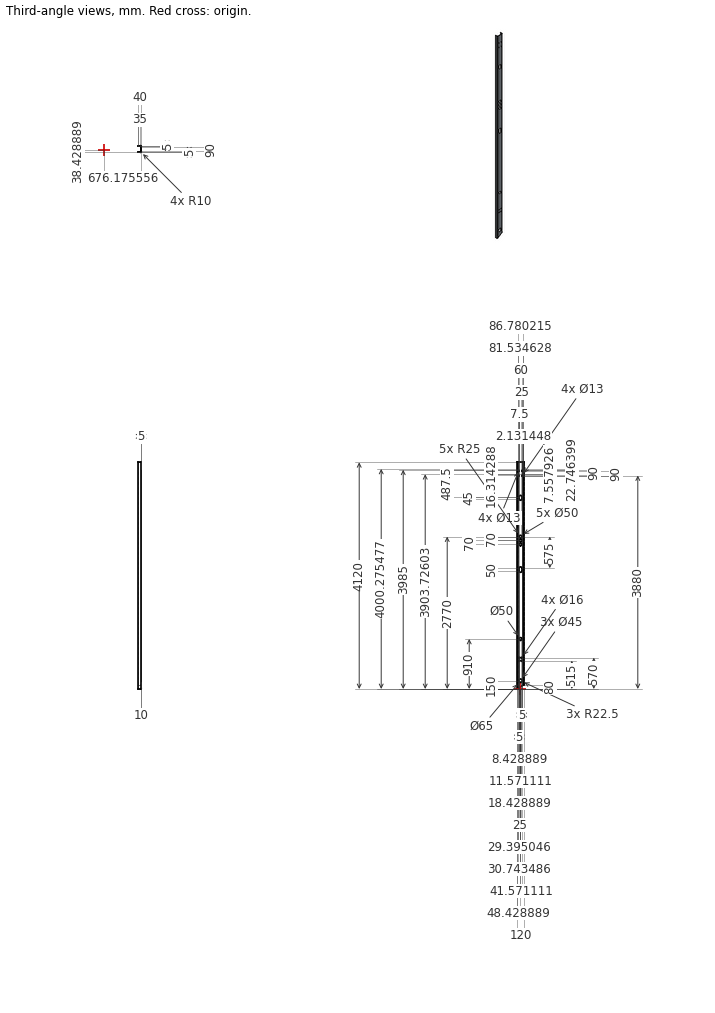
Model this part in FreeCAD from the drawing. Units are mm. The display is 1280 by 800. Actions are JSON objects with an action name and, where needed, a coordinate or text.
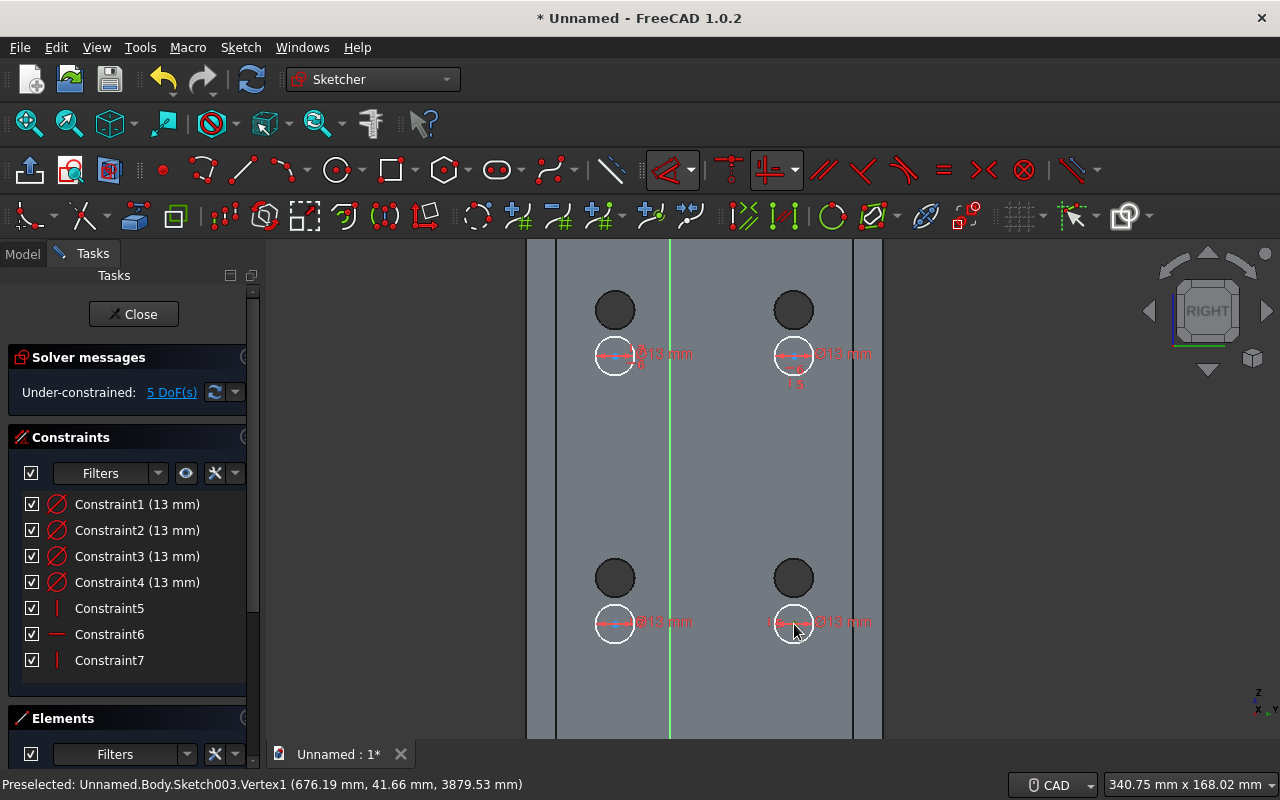
{"action": "left_click", "coordinate": [615, 624]}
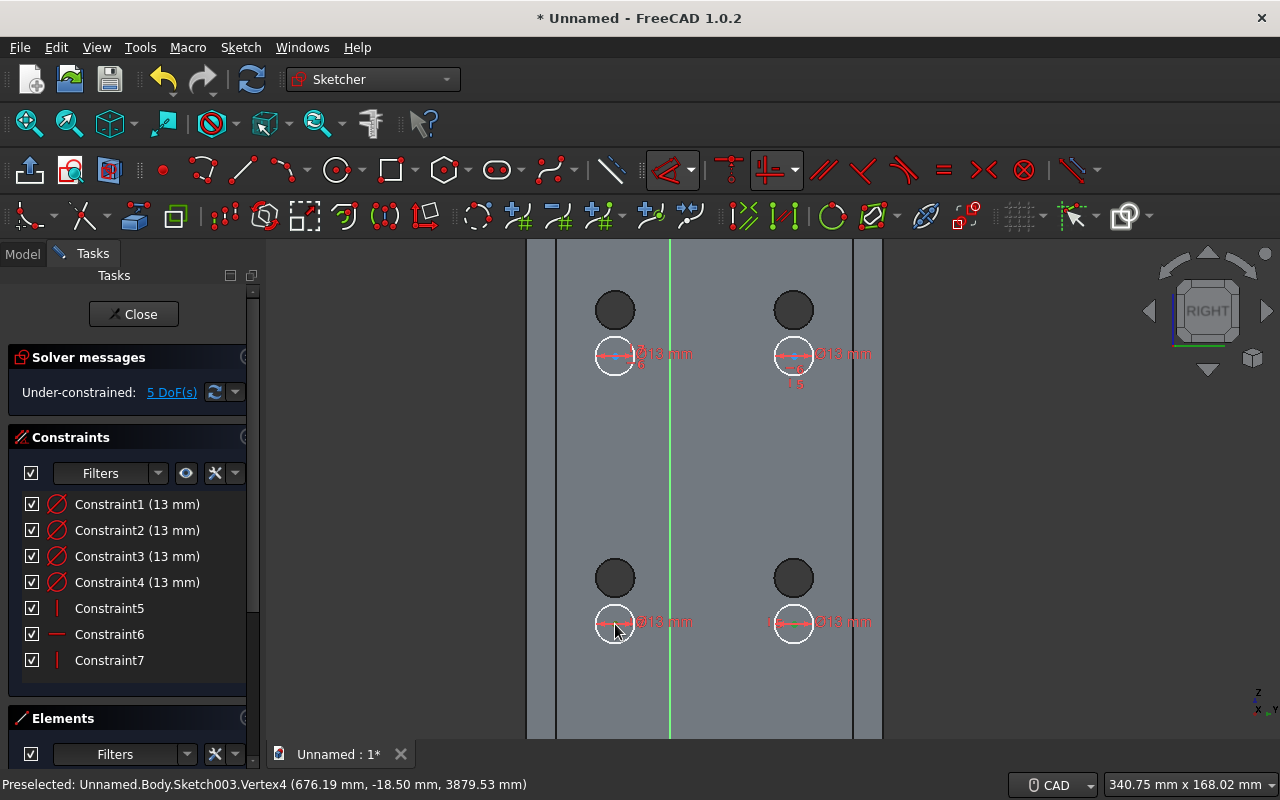
{"action": "left_click", "coordinate": [798, 170]}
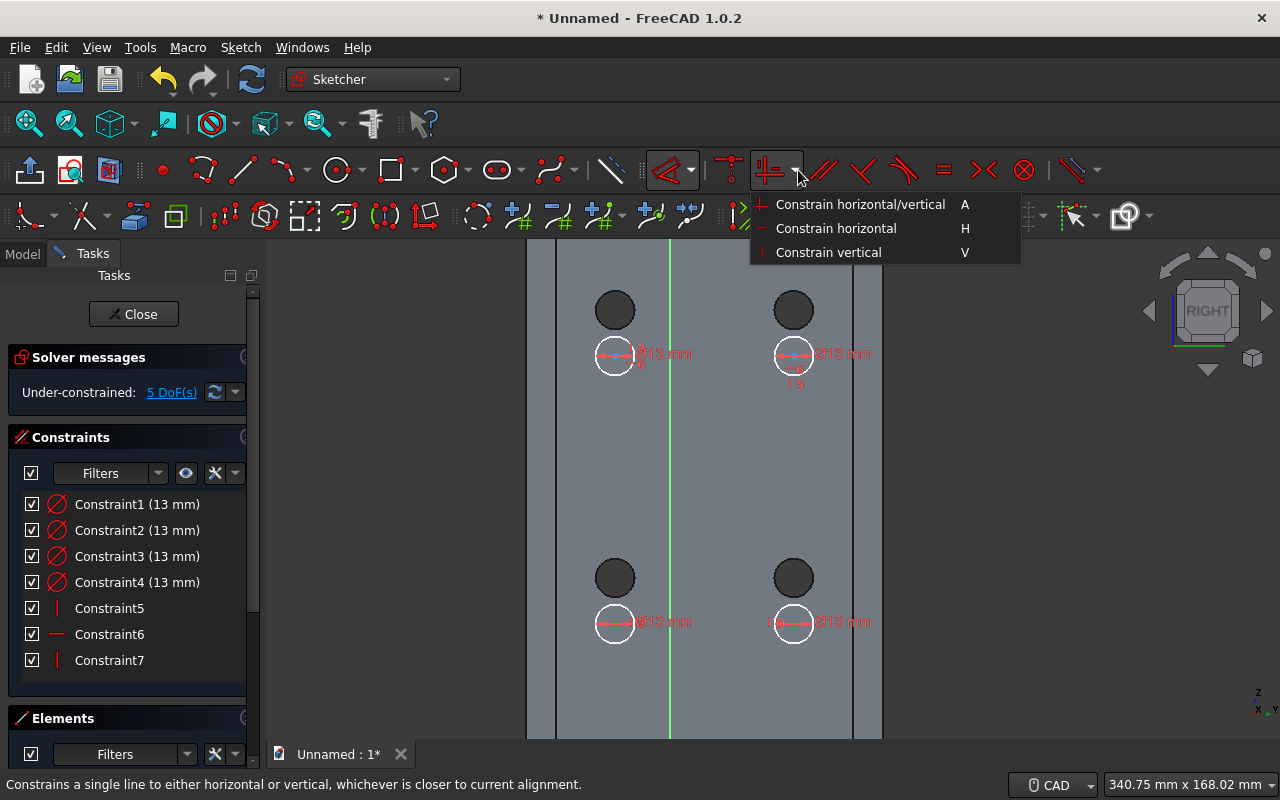
{"action": "left_click", "coordinate": [886, 228]}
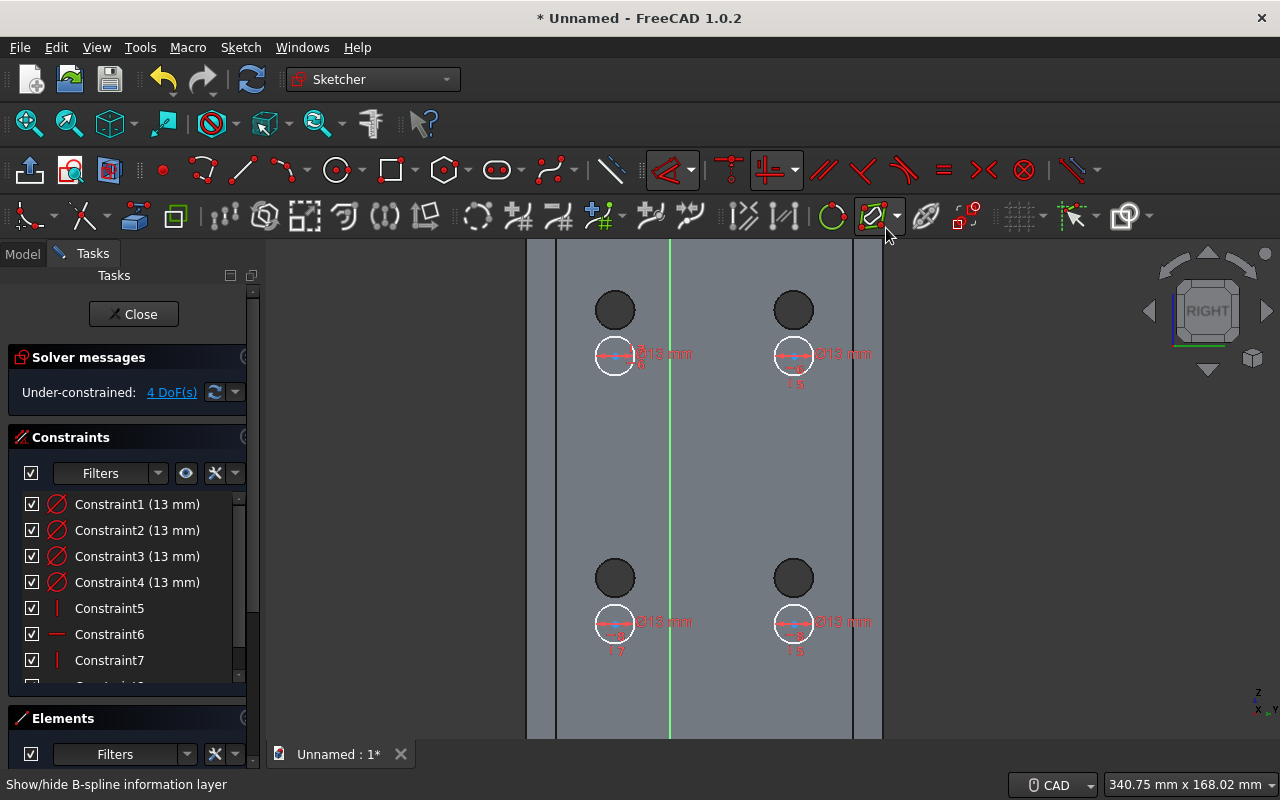
{"action": "left_click", "coordinate": [794, 624]}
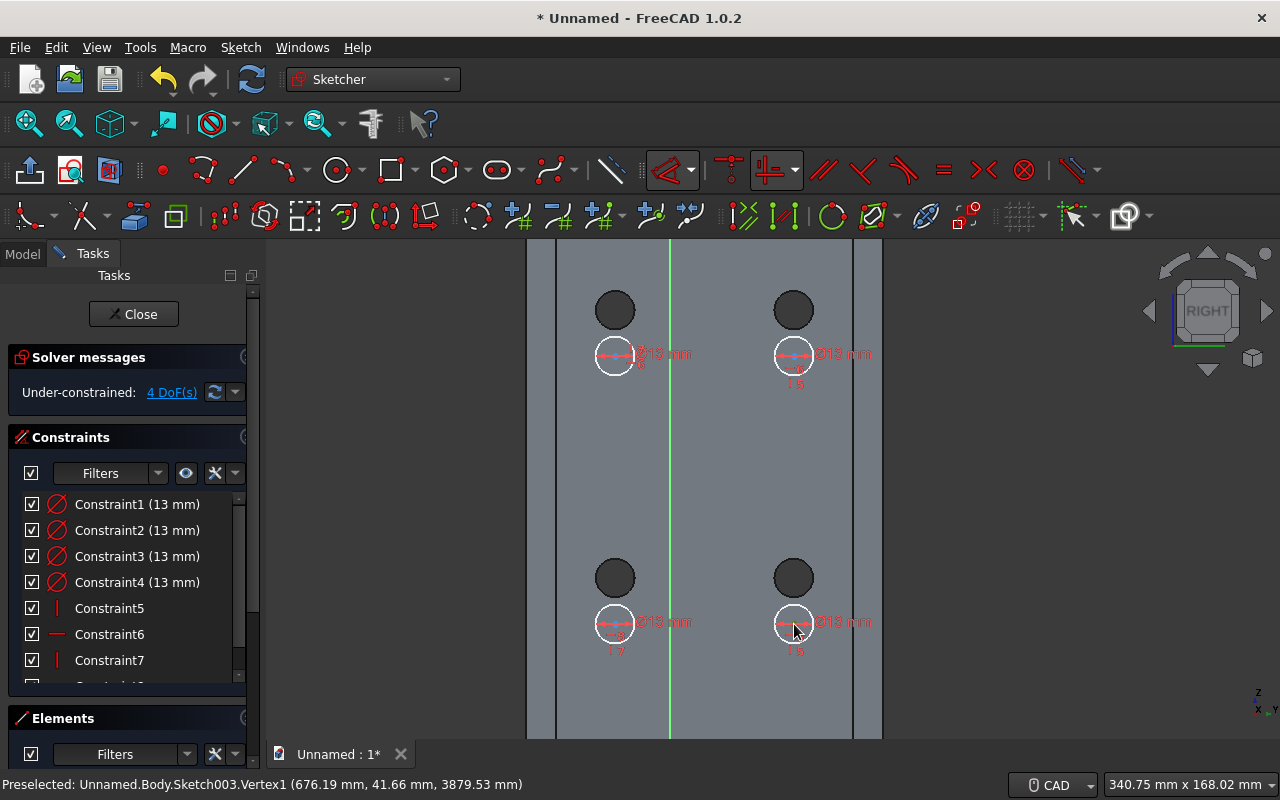
{"action": "left_click", "coordinate": [794, 356]}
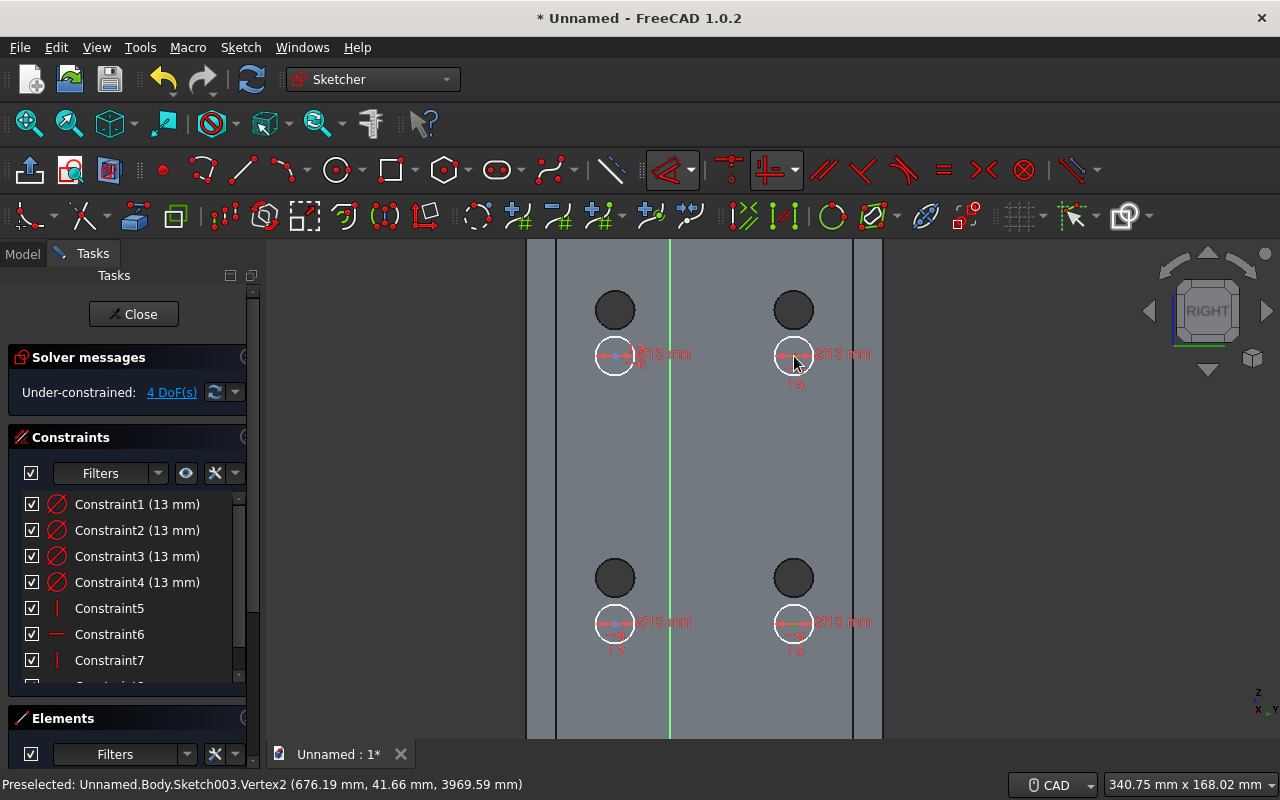
{"action": "left_click", "coordinate": [694, 170]}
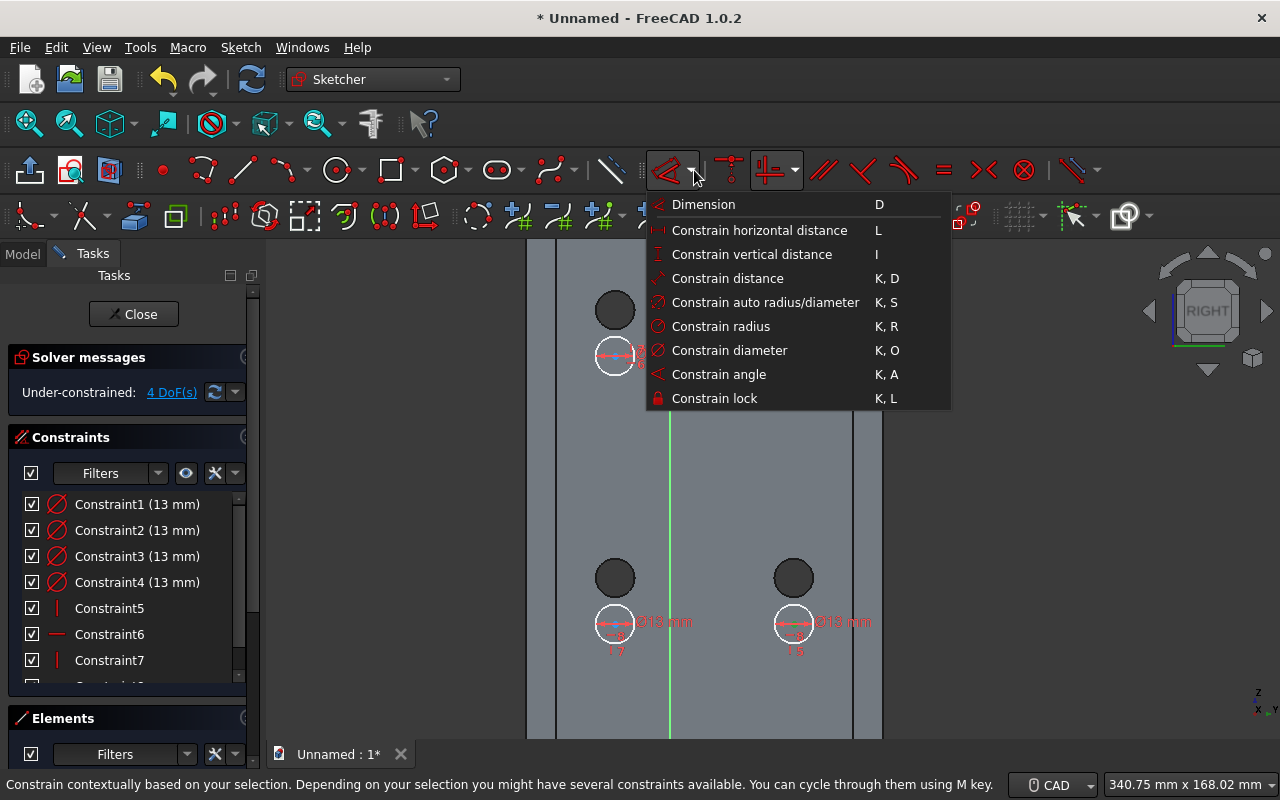
{"action": "left_click", "coordinate": [799, 254]}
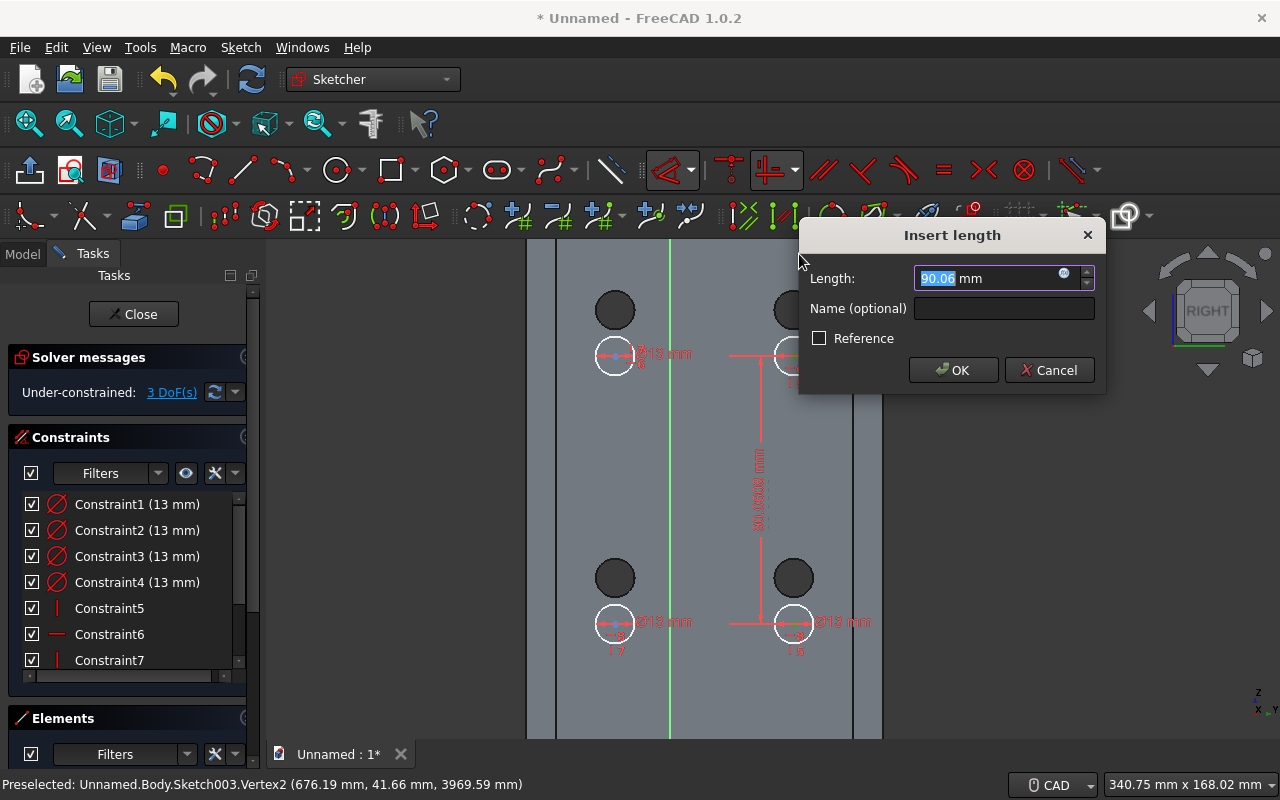
{"action": "type", "text": "90"}
{"action": "key", "text": "Return"}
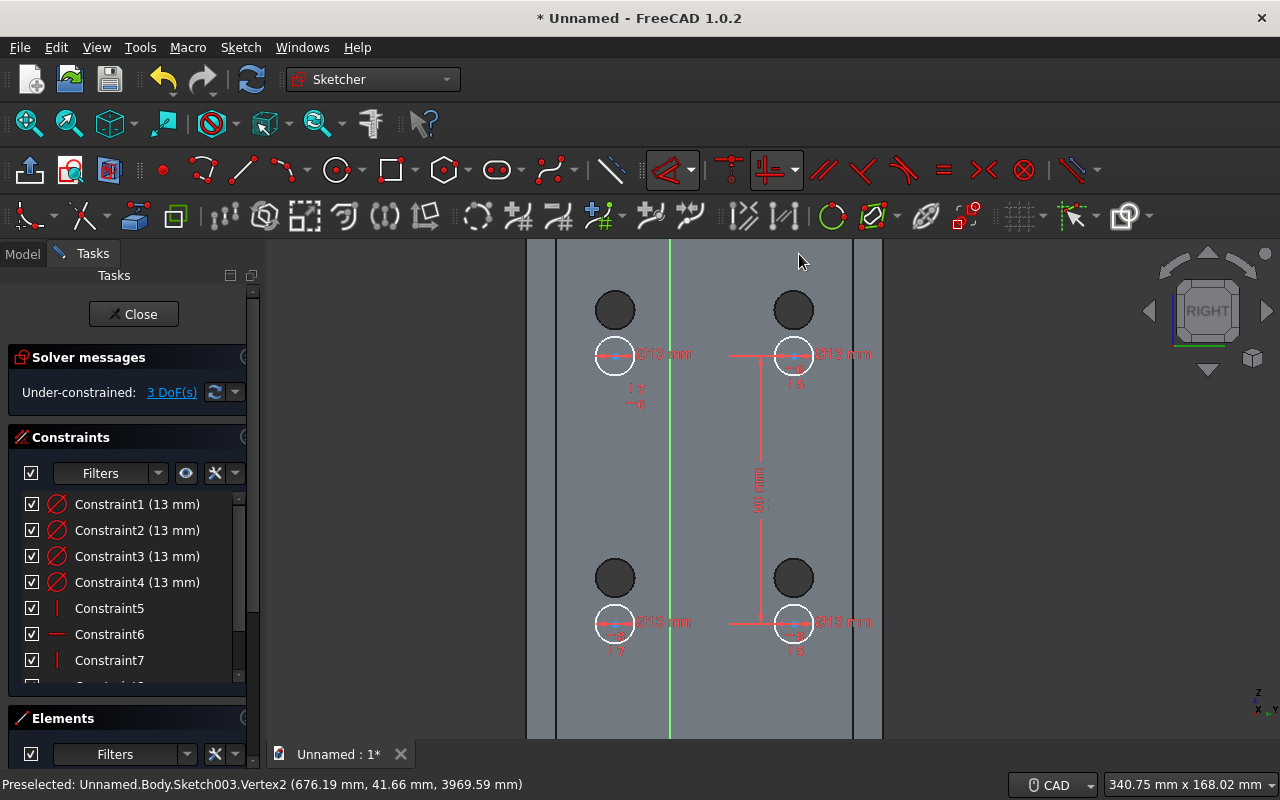
{"action": "left_click", "coordinate": [794, 356]}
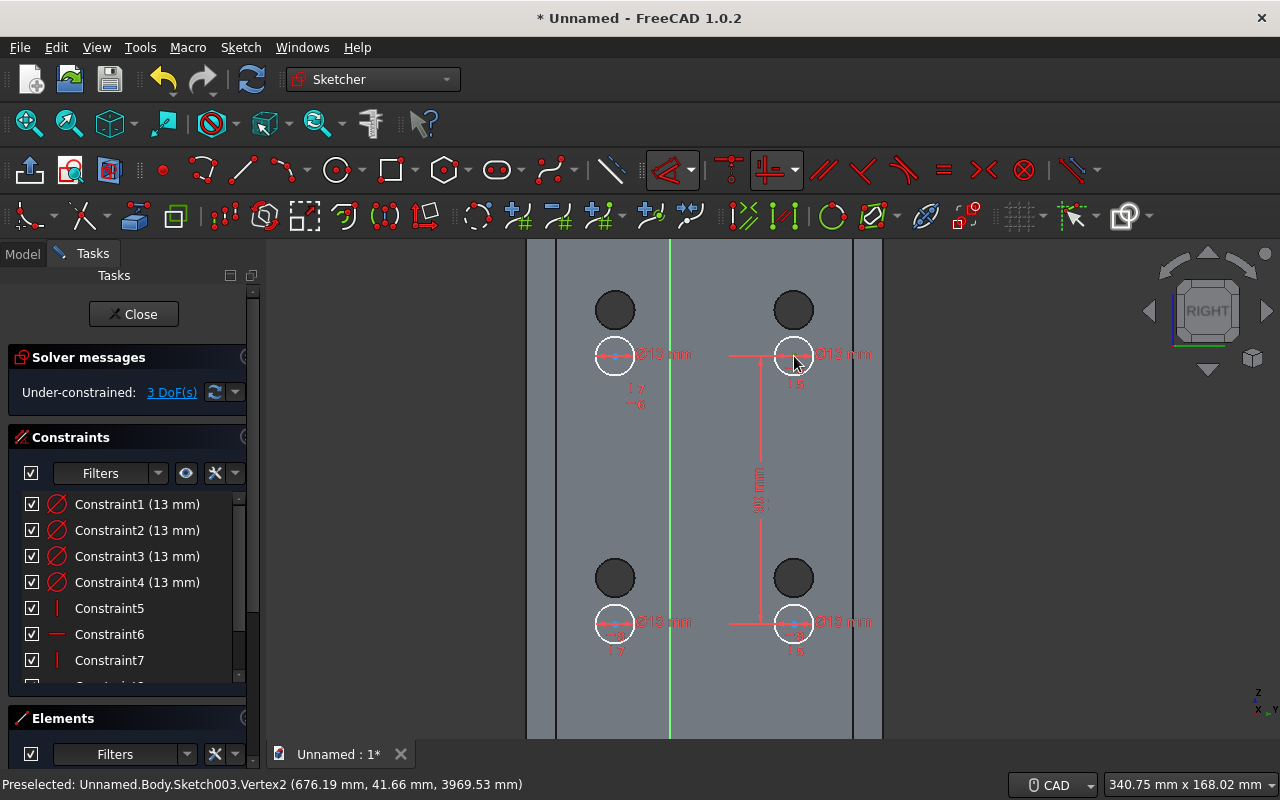
{"action": "left_click", "coordinate": [615, 356]}